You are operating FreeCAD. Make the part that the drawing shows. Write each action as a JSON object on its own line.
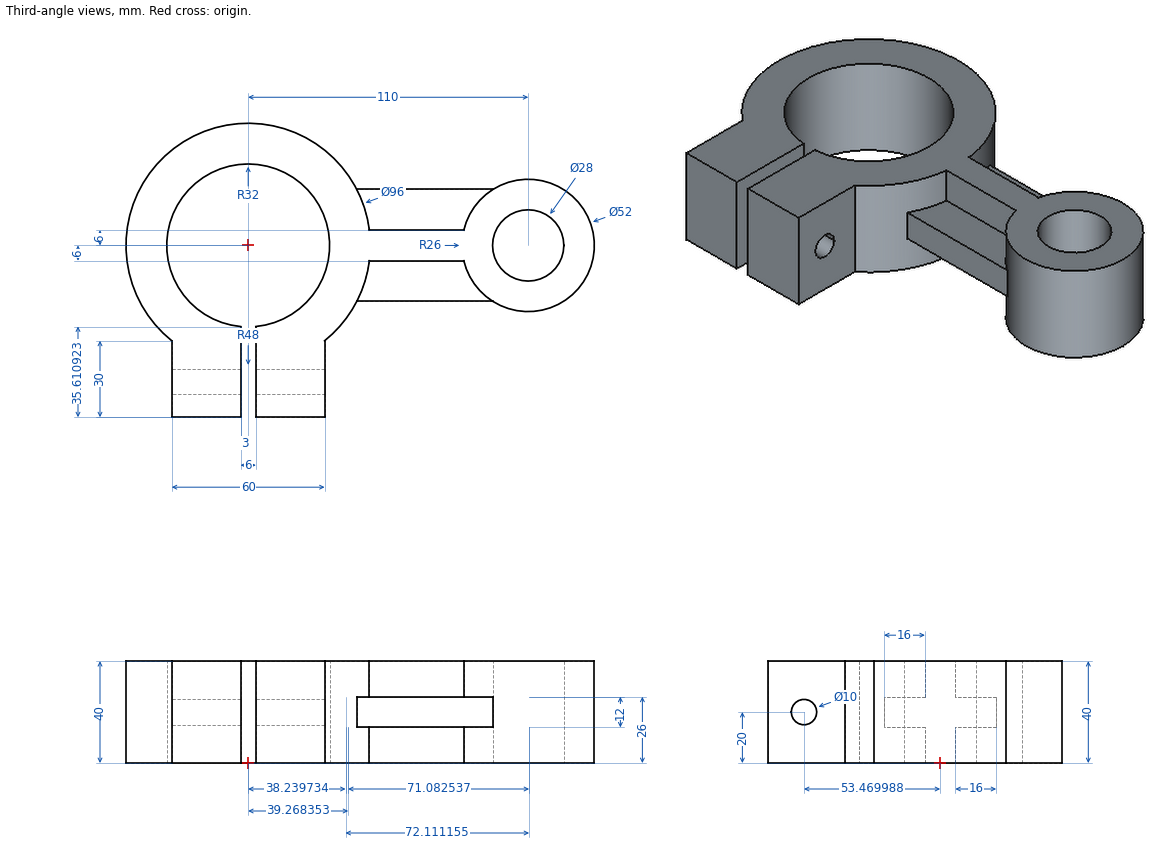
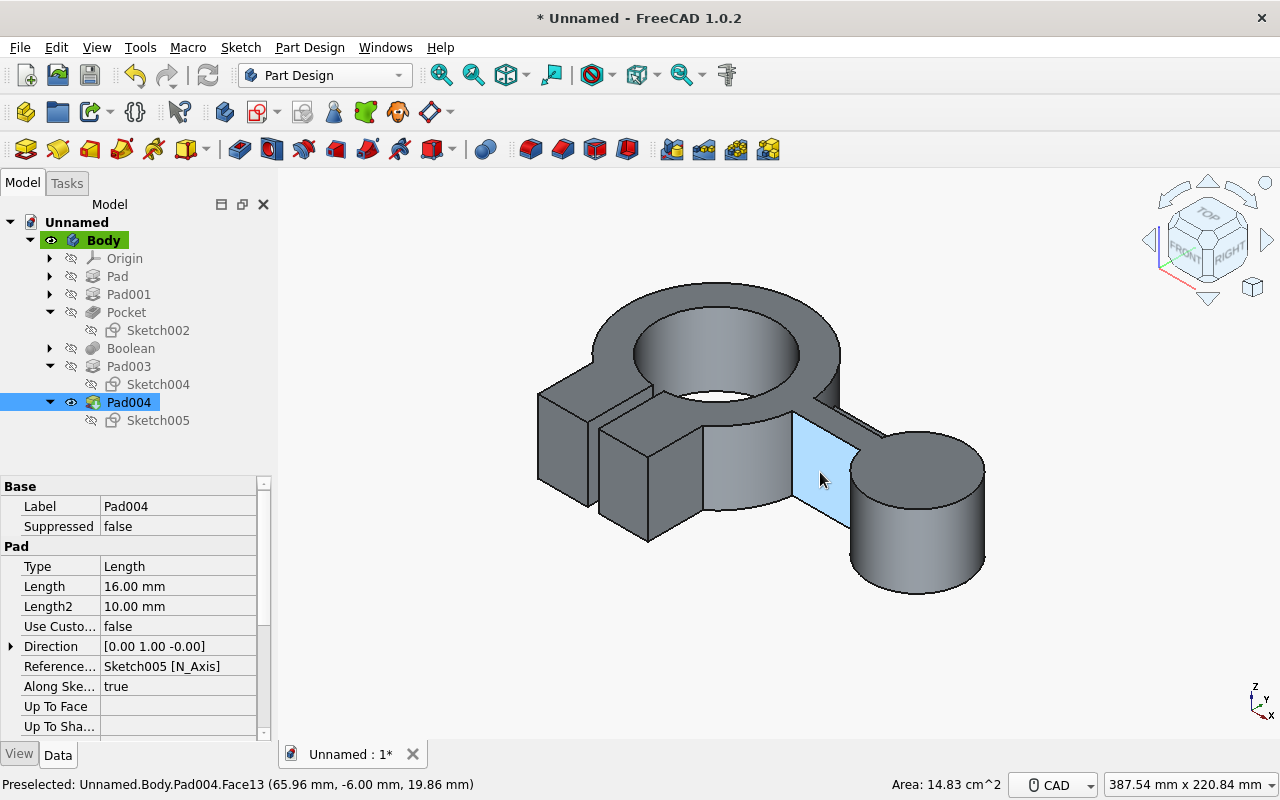
{"action": "left_click", "coordinate": [258, 112]}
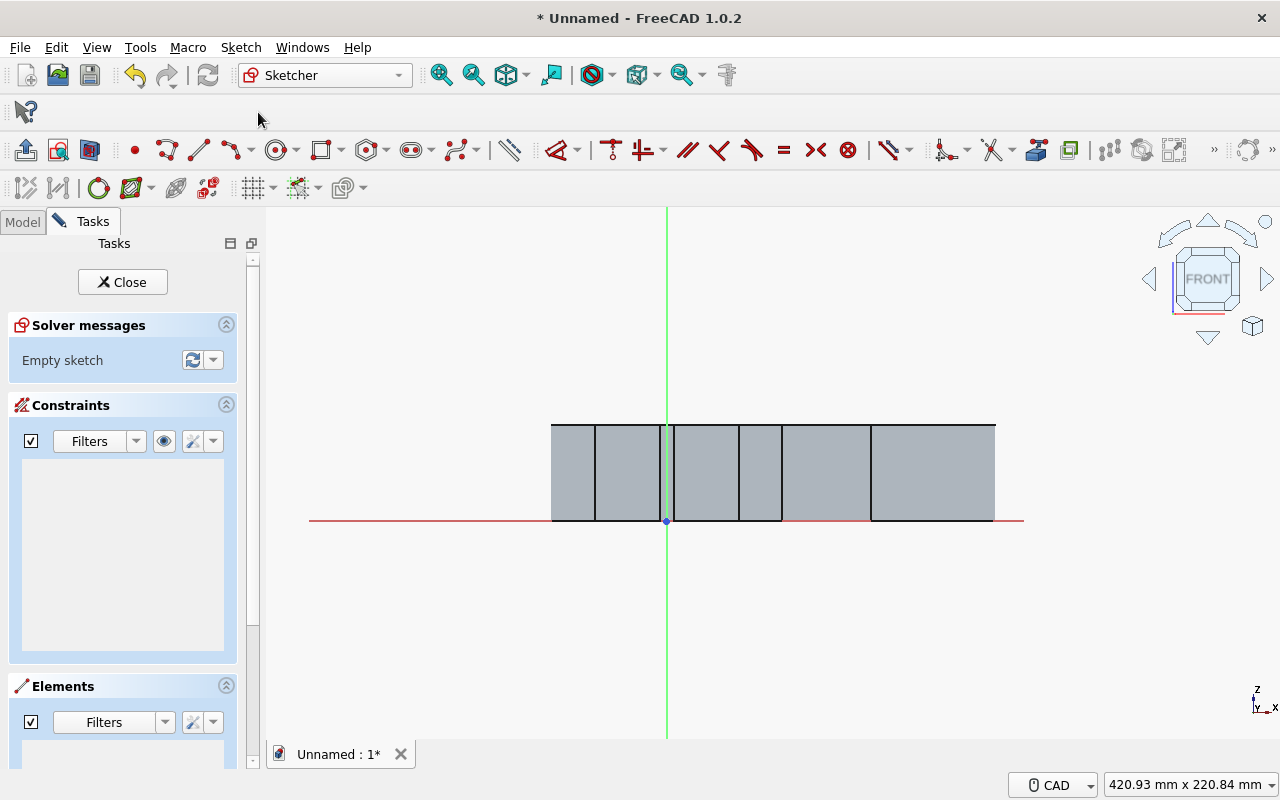
{"action": "left_click", "coordinate": [90, 150]}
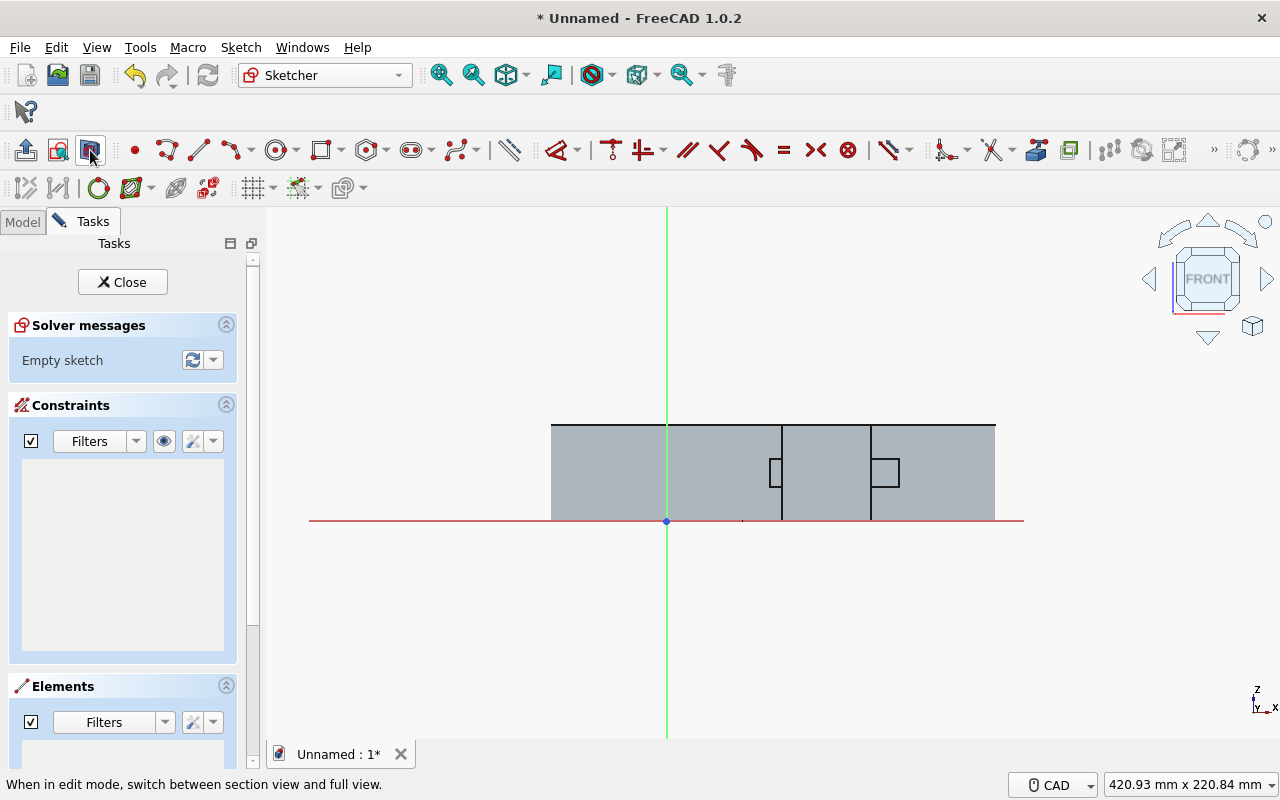
{"action": "scroll", "coordinate": [878, 504], "scroll_direction": "up", "scroll_amount": 4}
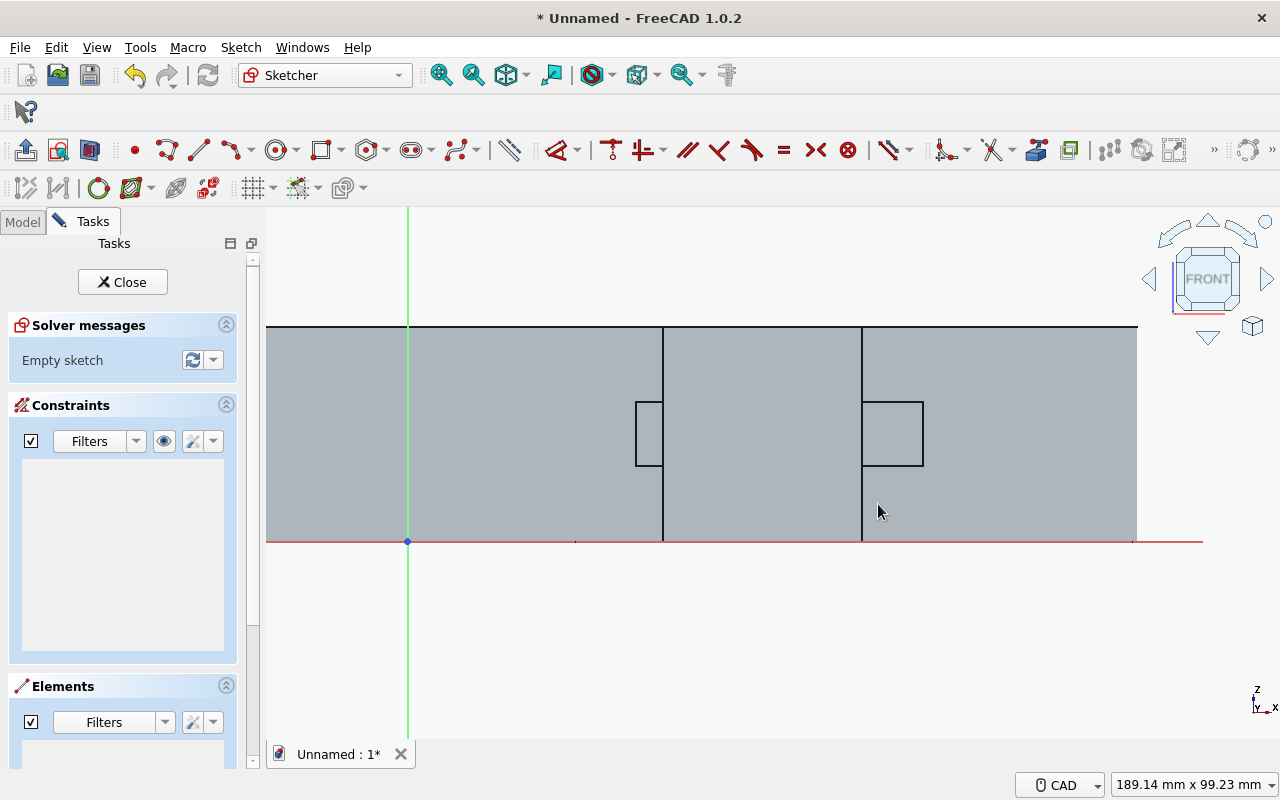
{"action": "left_click", "coordinate": [322, 150]}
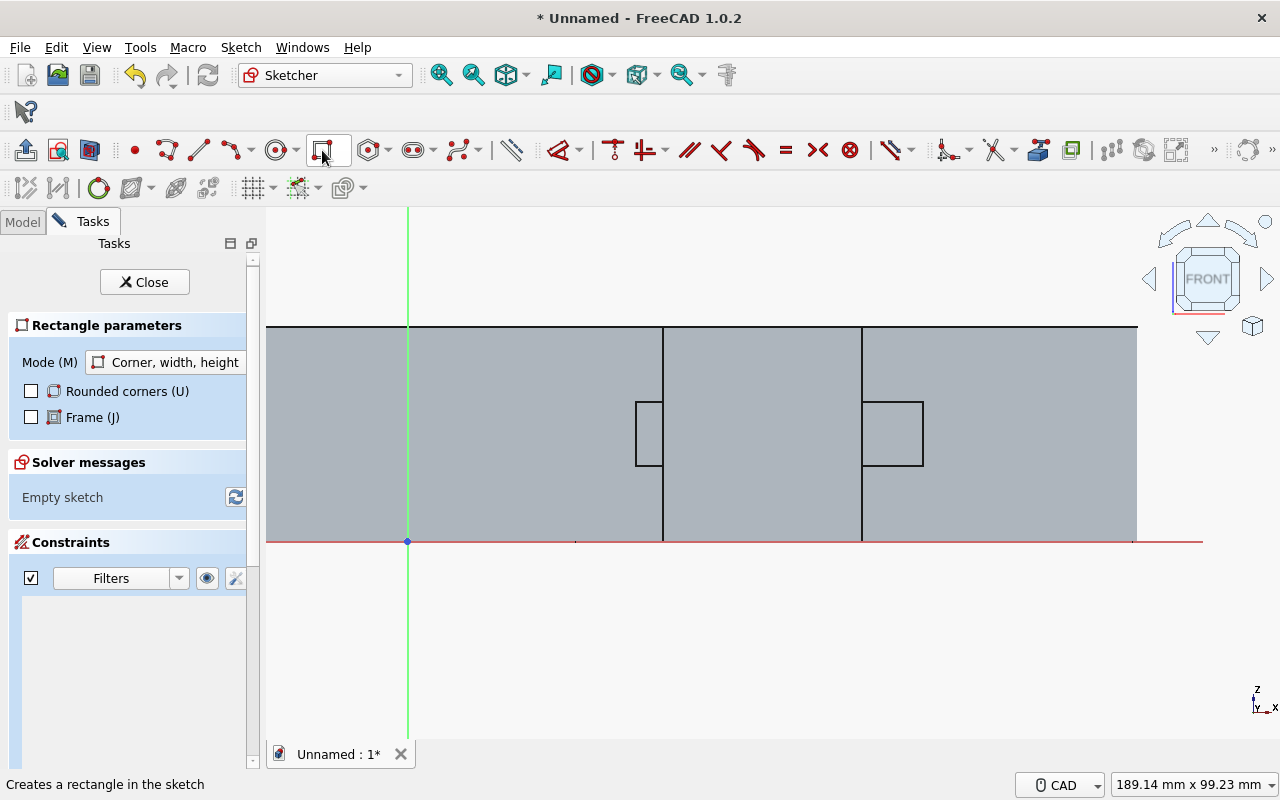
{"action": "left_click", "coordinate": [613, 402]}
{"action": "left_click", "coordinate": [999, 466]}
{"action": "key", "text": "Escape"}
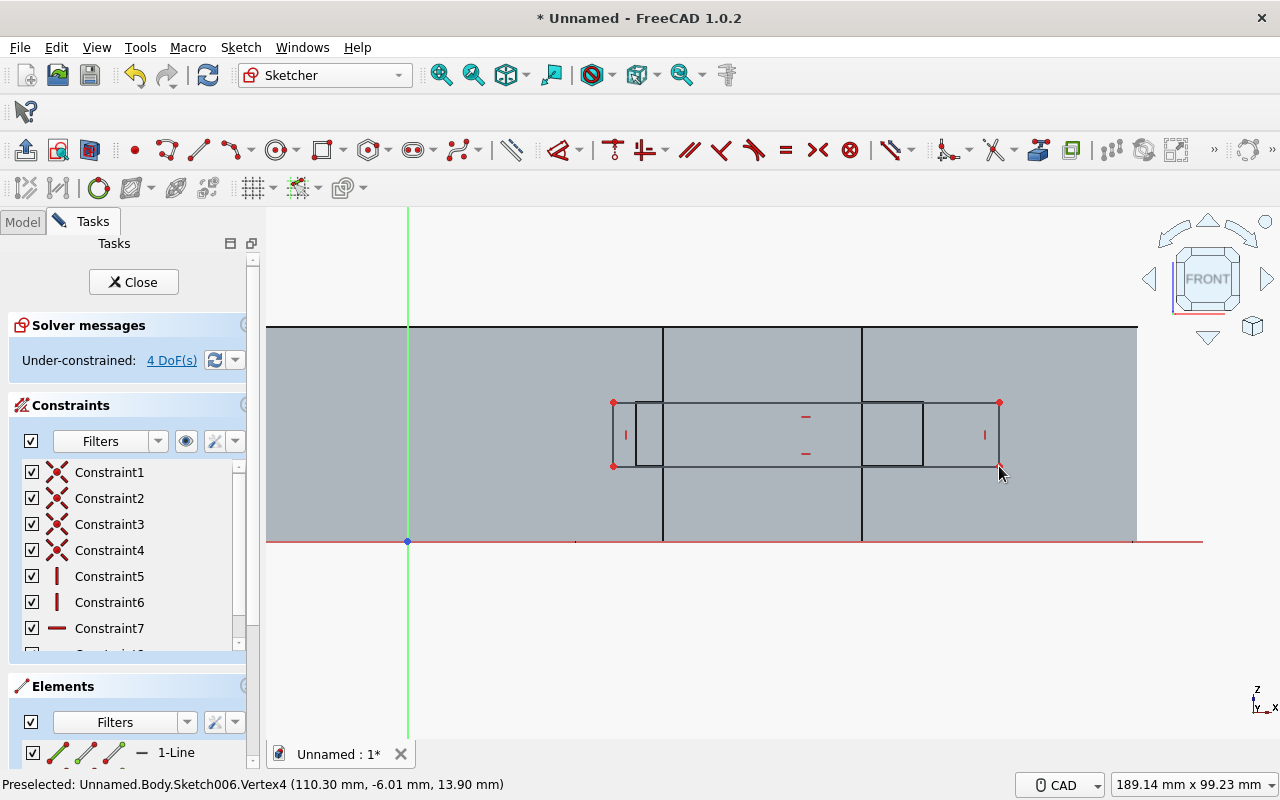
{"action": "left_click", "coordinate": [558, 150]}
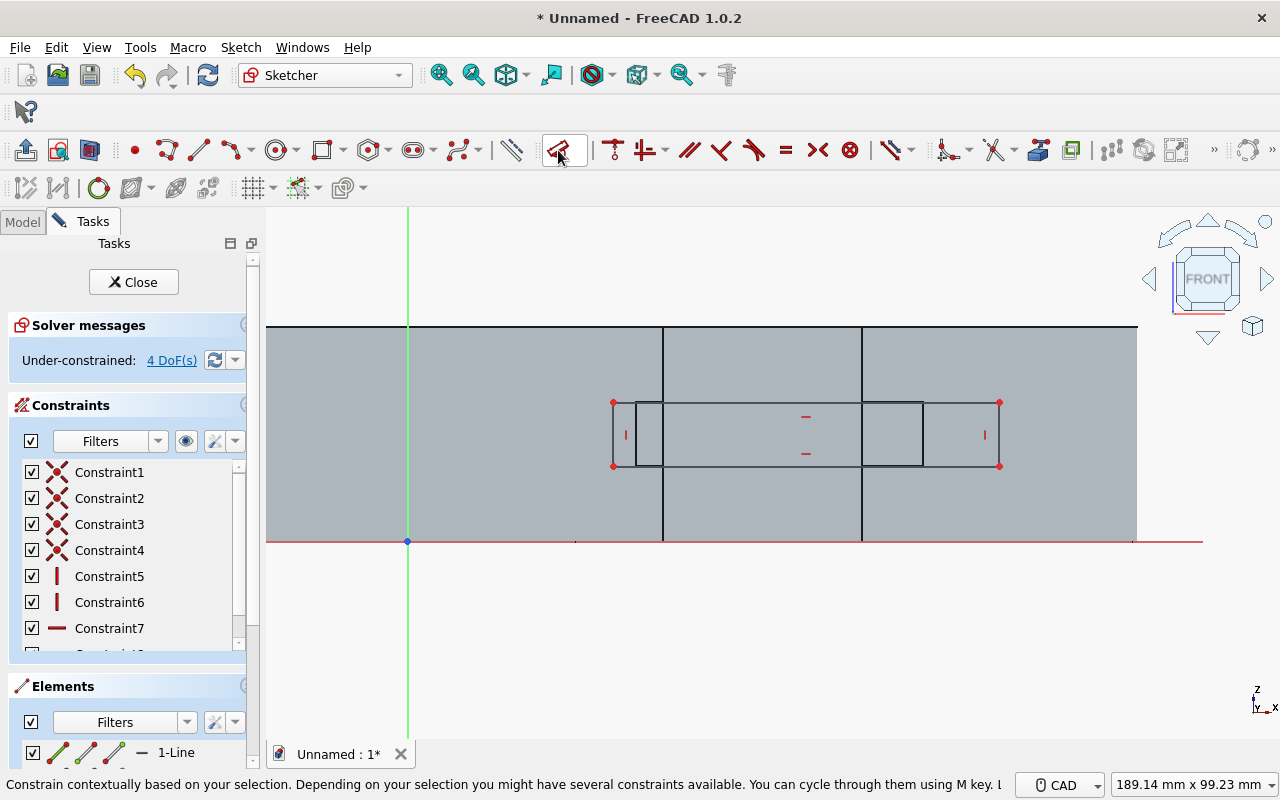
{"action": "left_click", "coordinate": [613, 422]}
{"action": "left_click", "coordinate": [579, 435]}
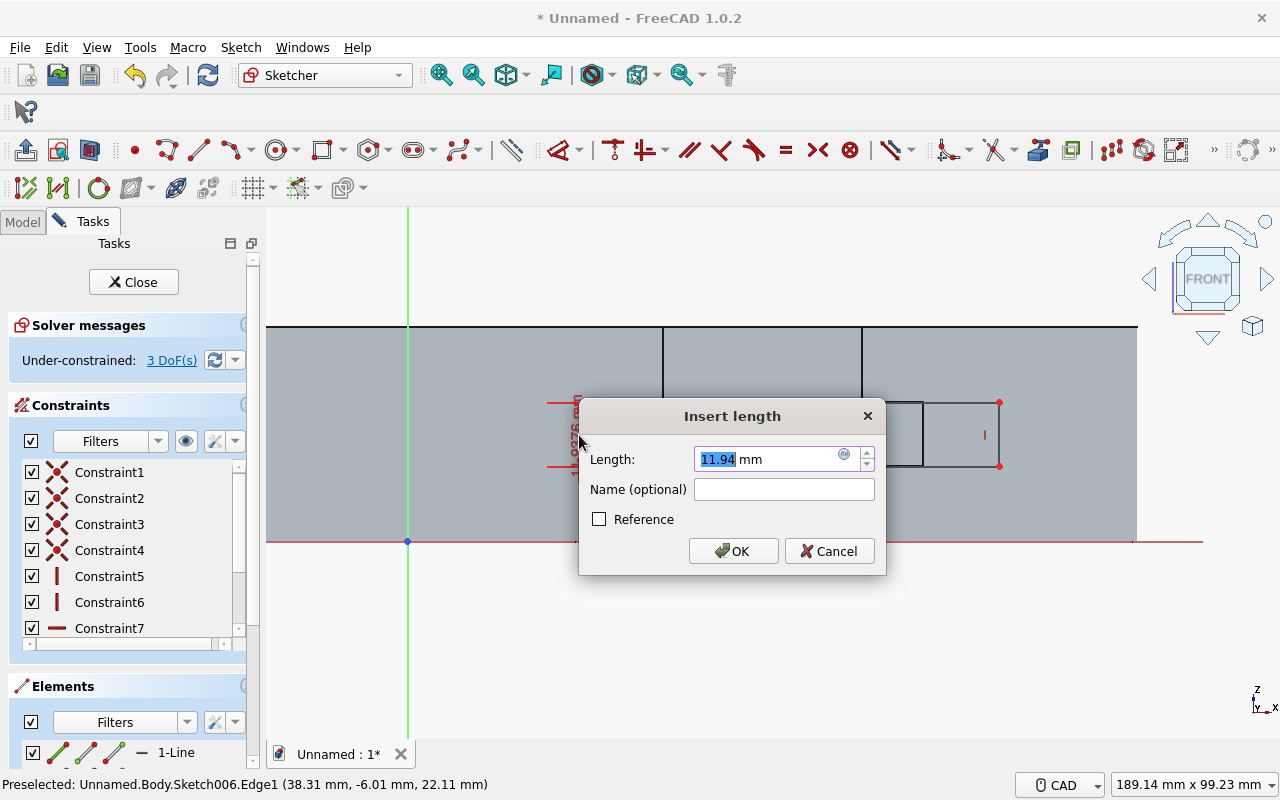
{"action": "type", "text": "12"}
{"action": "key", "text": "Return"}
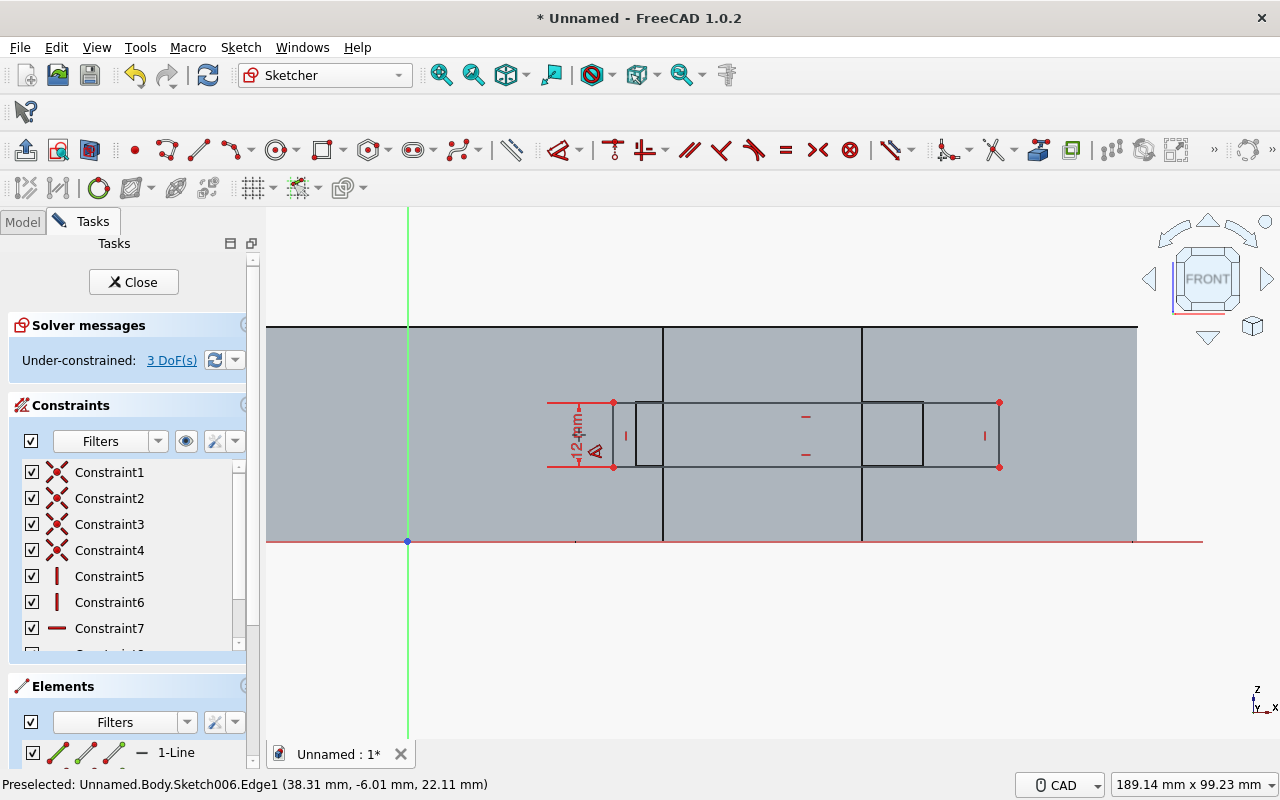
{"action": "left_click", "coordinate": [613, 403]}
{"action": "left_click", "coordinate": [374, 472]}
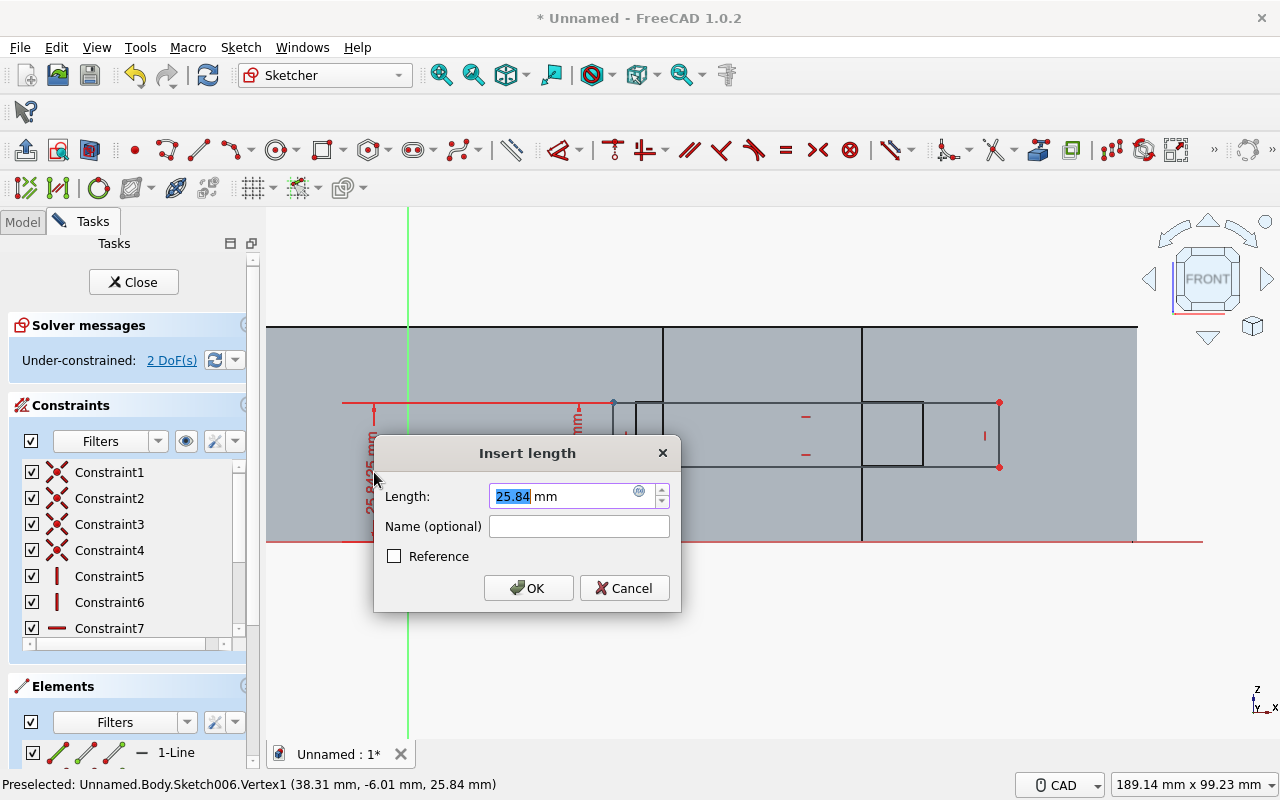
{"action": "type", "text": "26"}
{"action": "key", "text": "Return"}